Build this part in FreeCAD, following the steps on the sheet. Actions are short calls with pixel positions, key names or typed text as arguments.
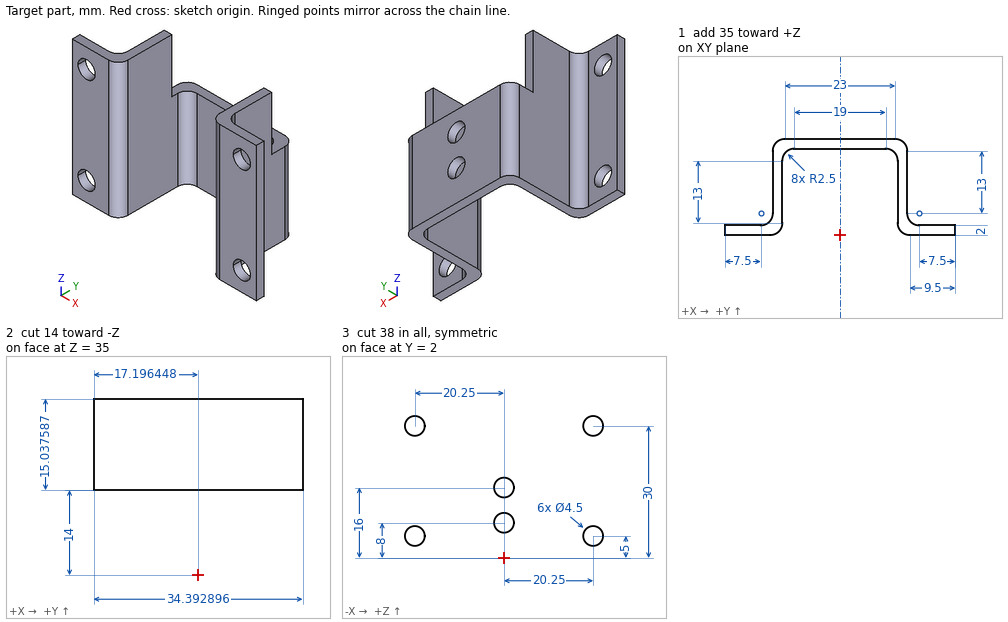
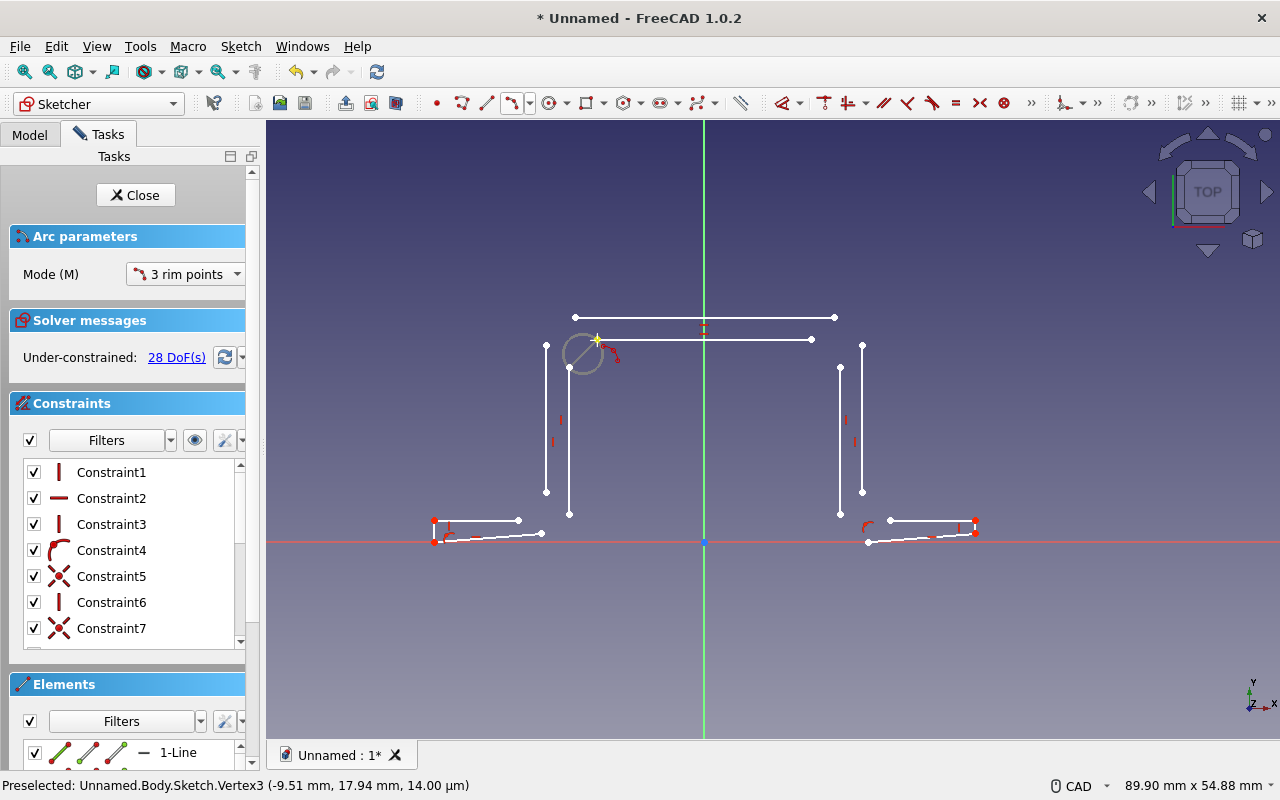
scroll(577, 348, up, 4)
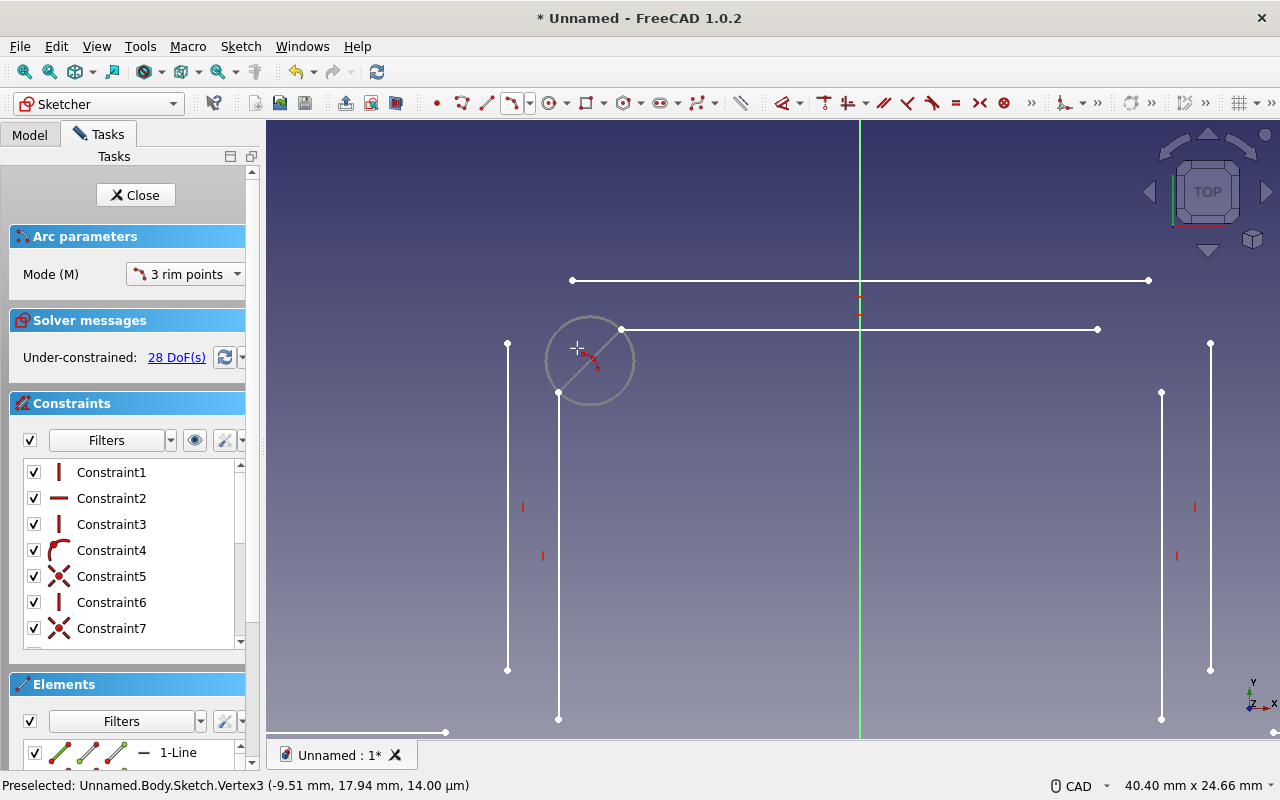
click(577, 347)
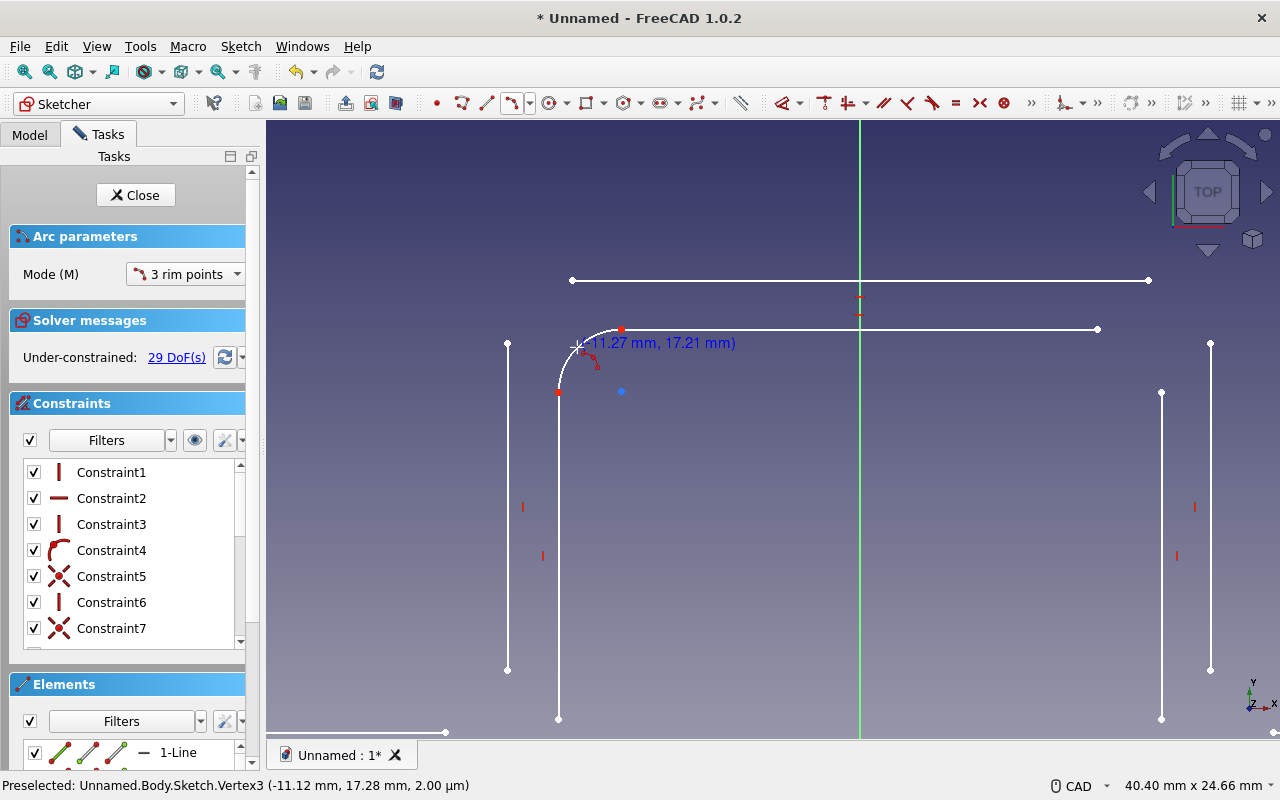
click(1097, 330)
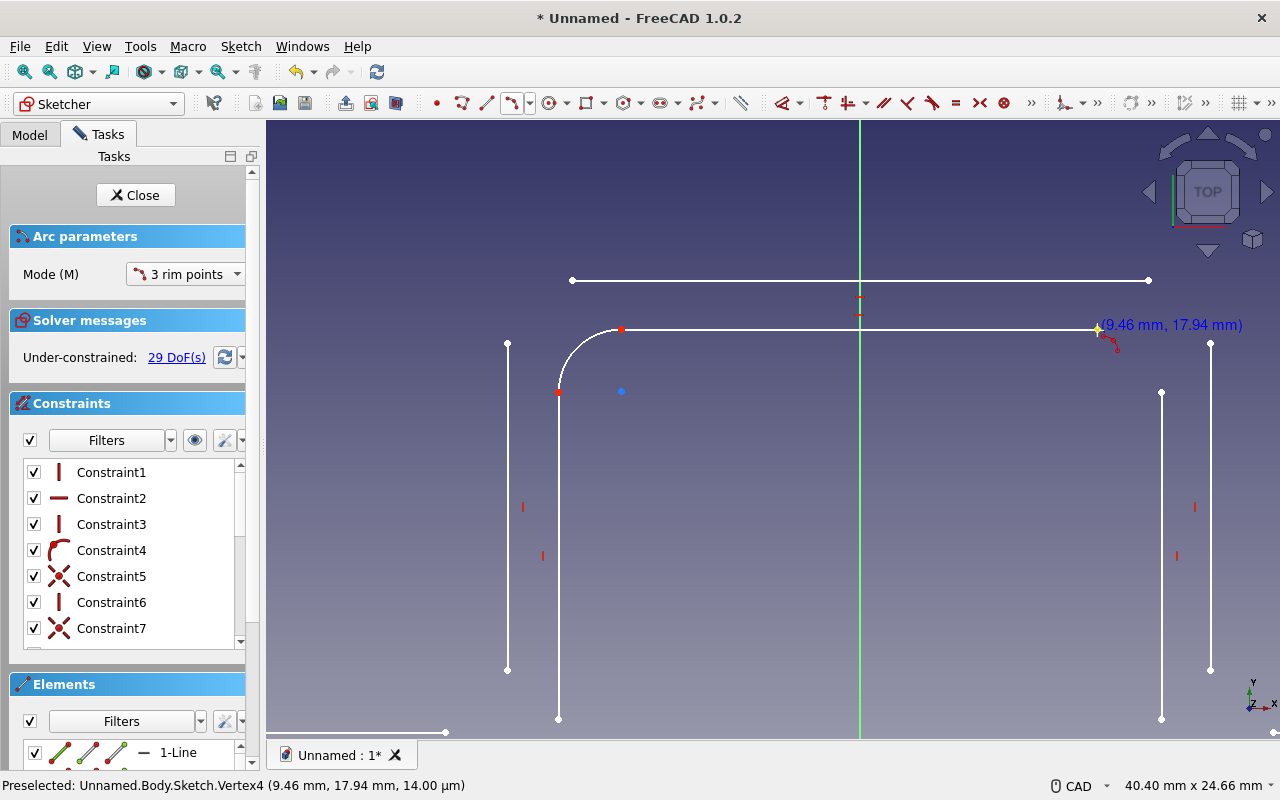
scroll(578, 348, down, 4)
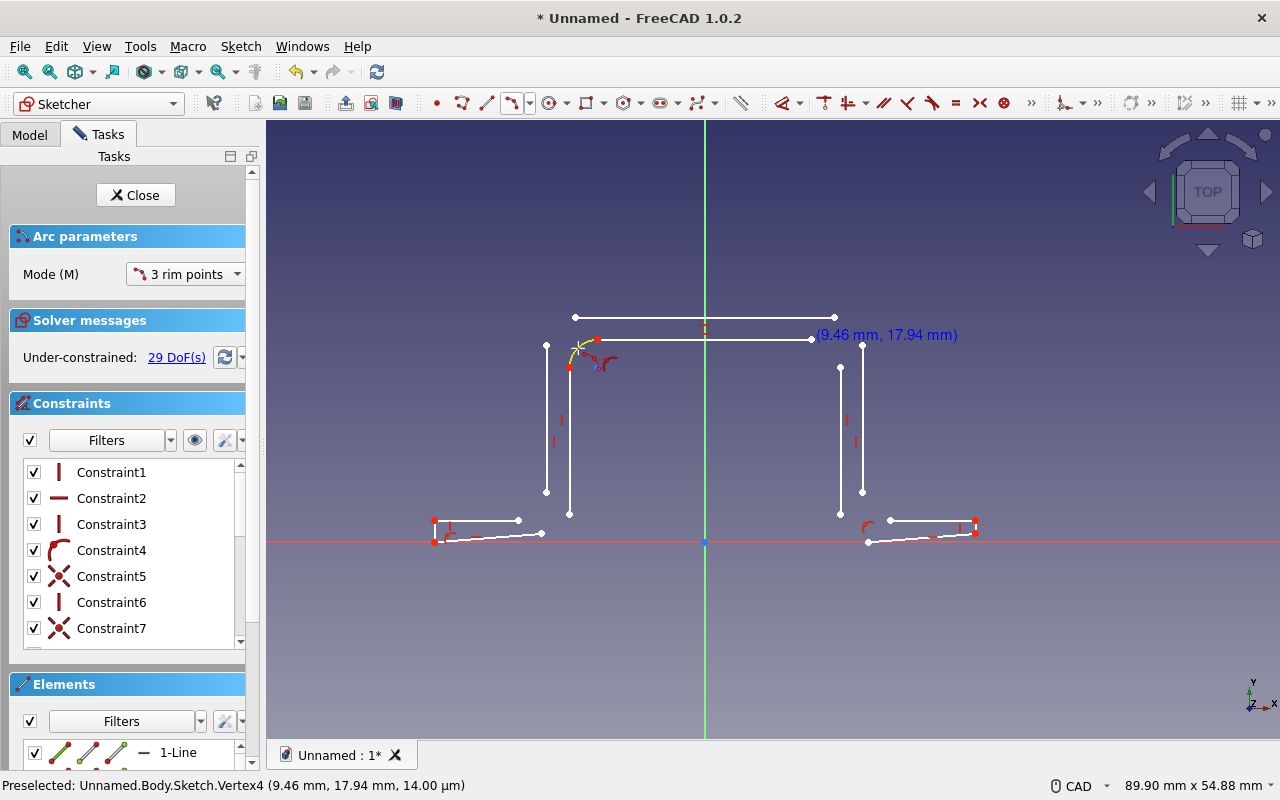
click(841, 368)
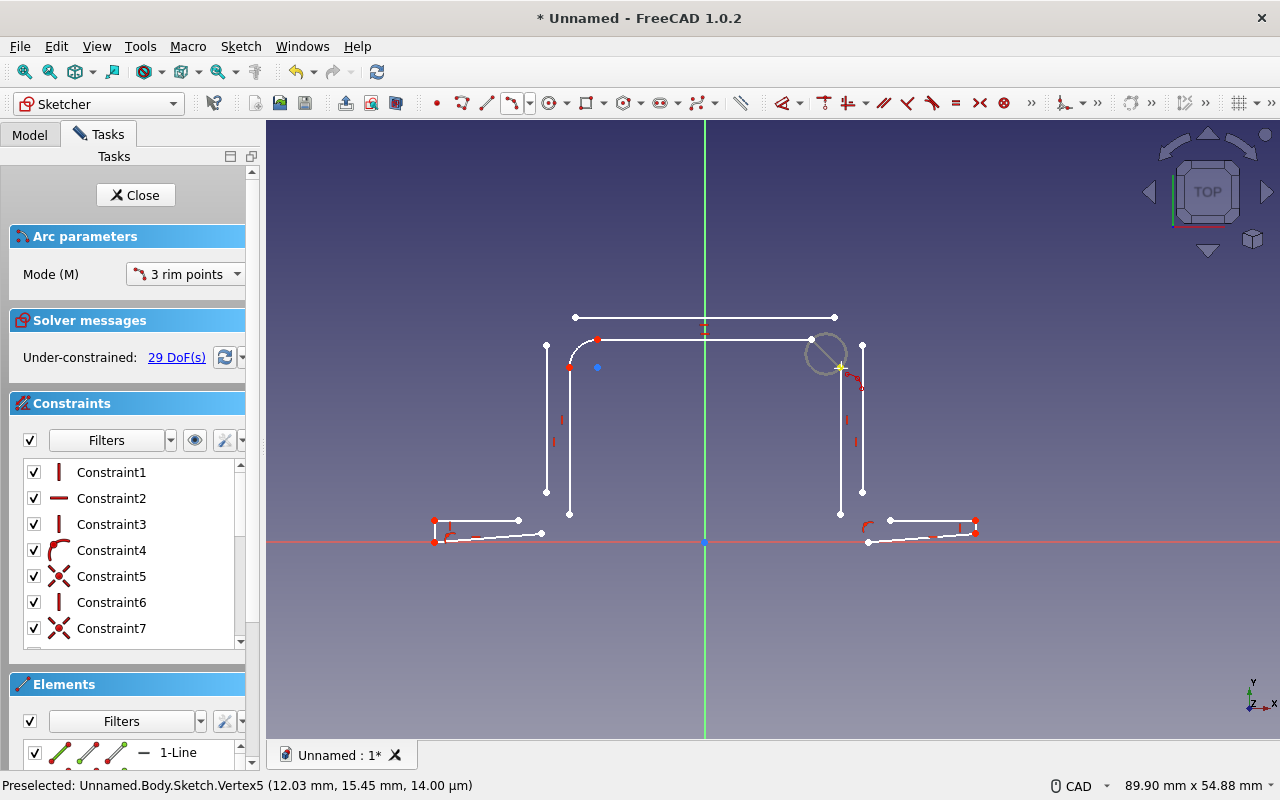
scroll(832, 348, up, 4)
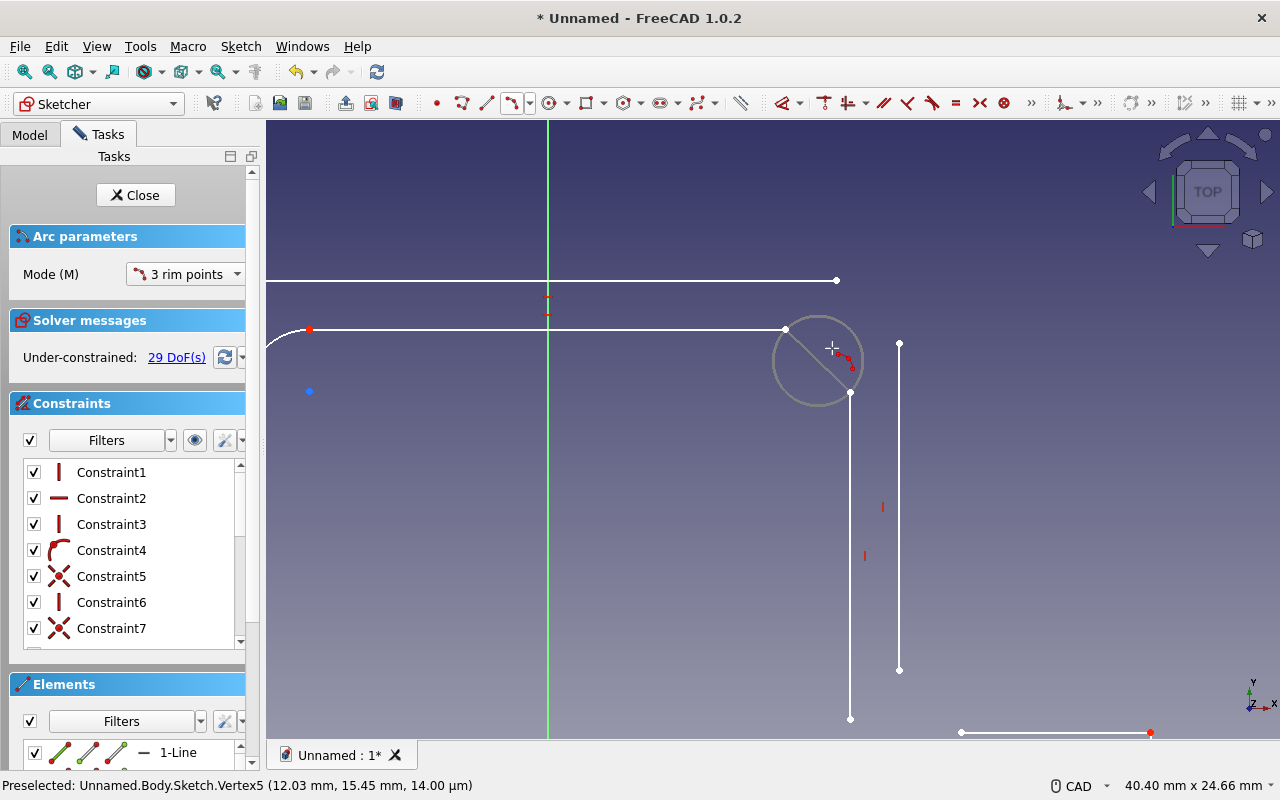
click(831, 347)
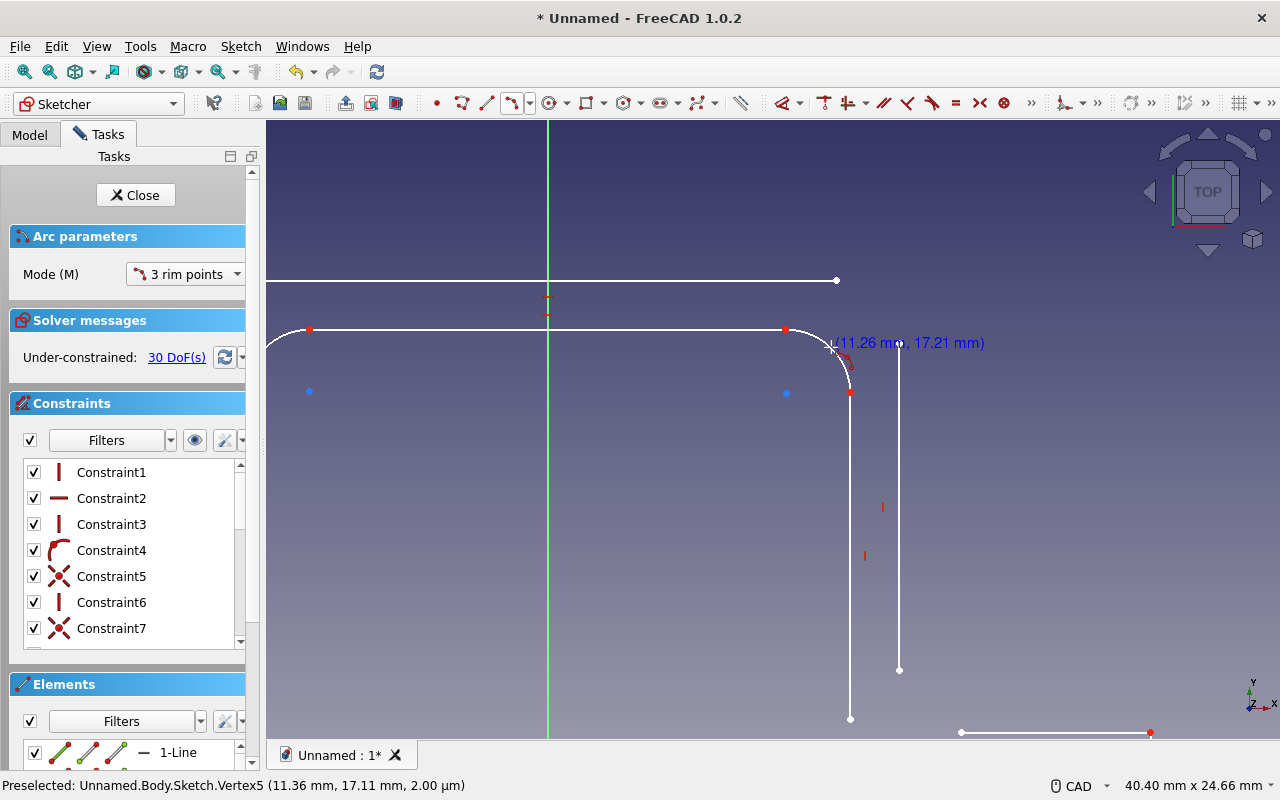
scroll(832, 348, down, 4)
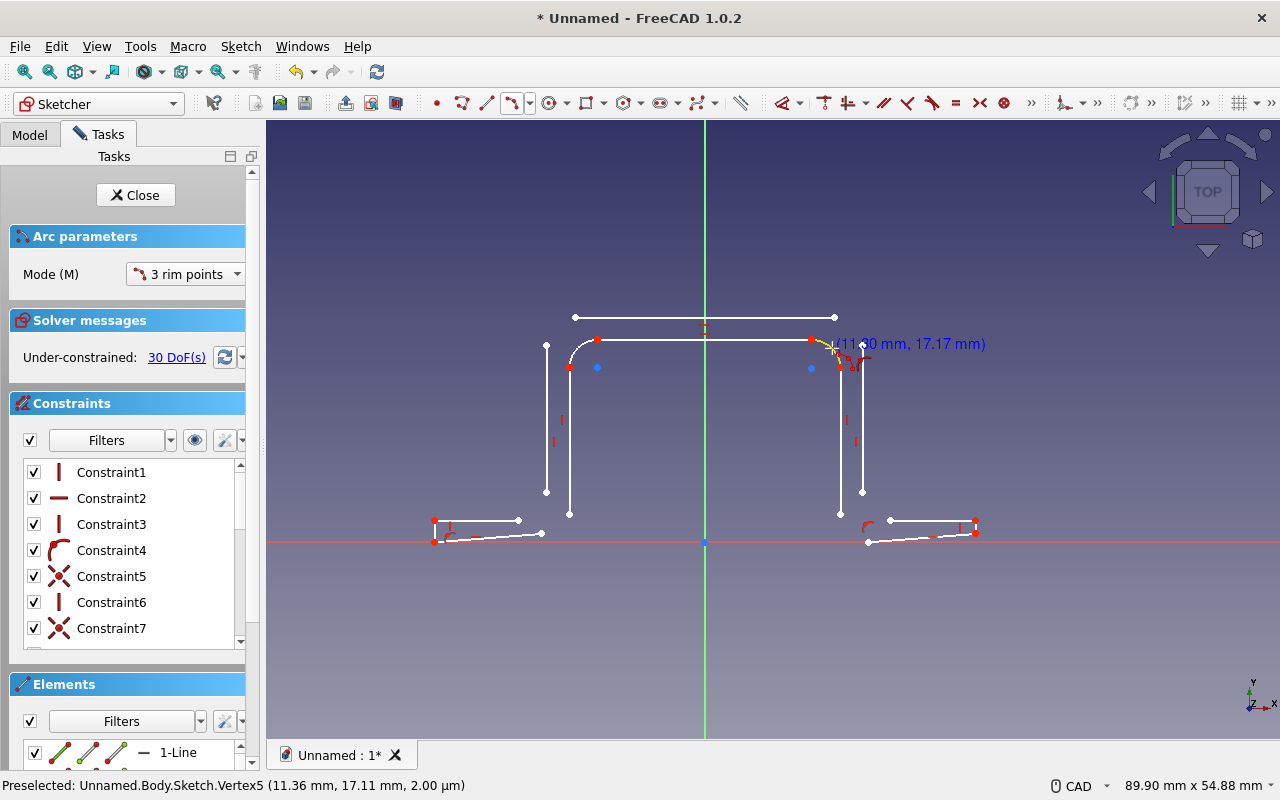
click(841, 515)
click(869, 542)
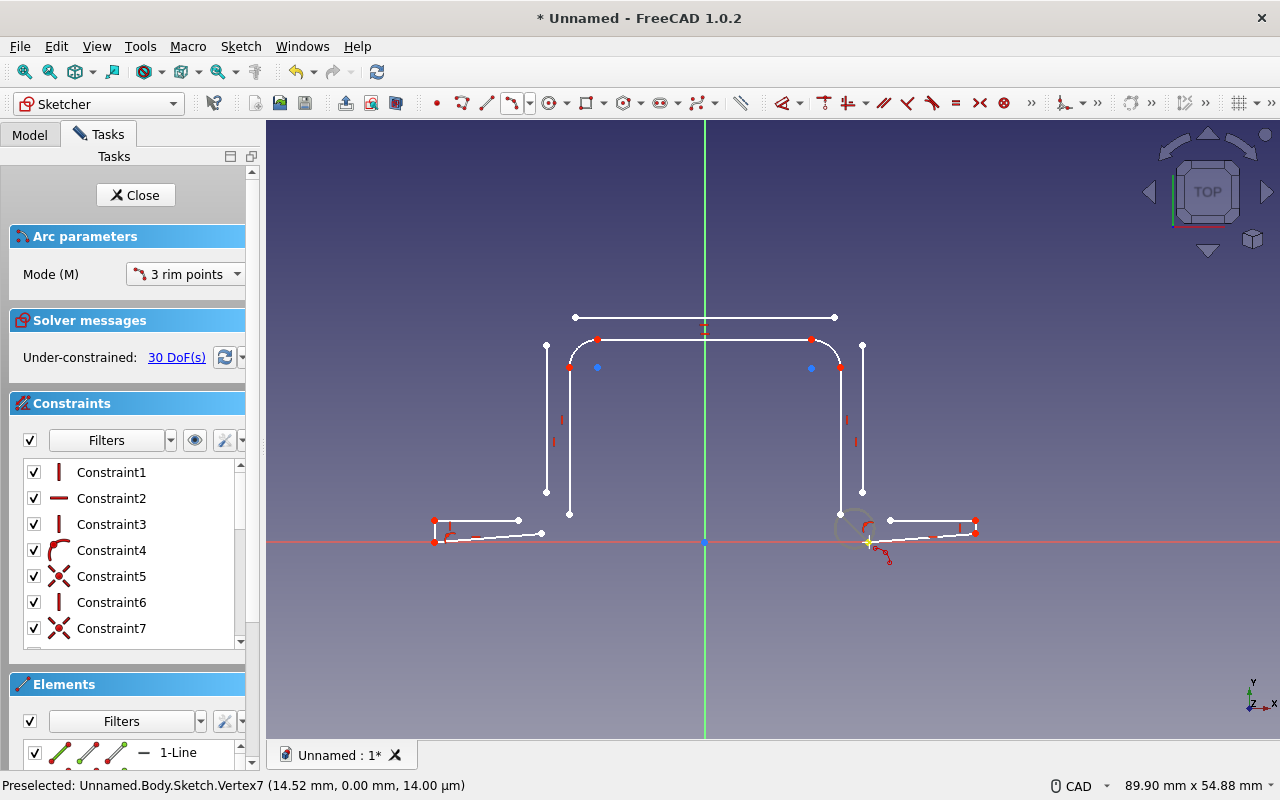
scroll(848, 534, up, 4)